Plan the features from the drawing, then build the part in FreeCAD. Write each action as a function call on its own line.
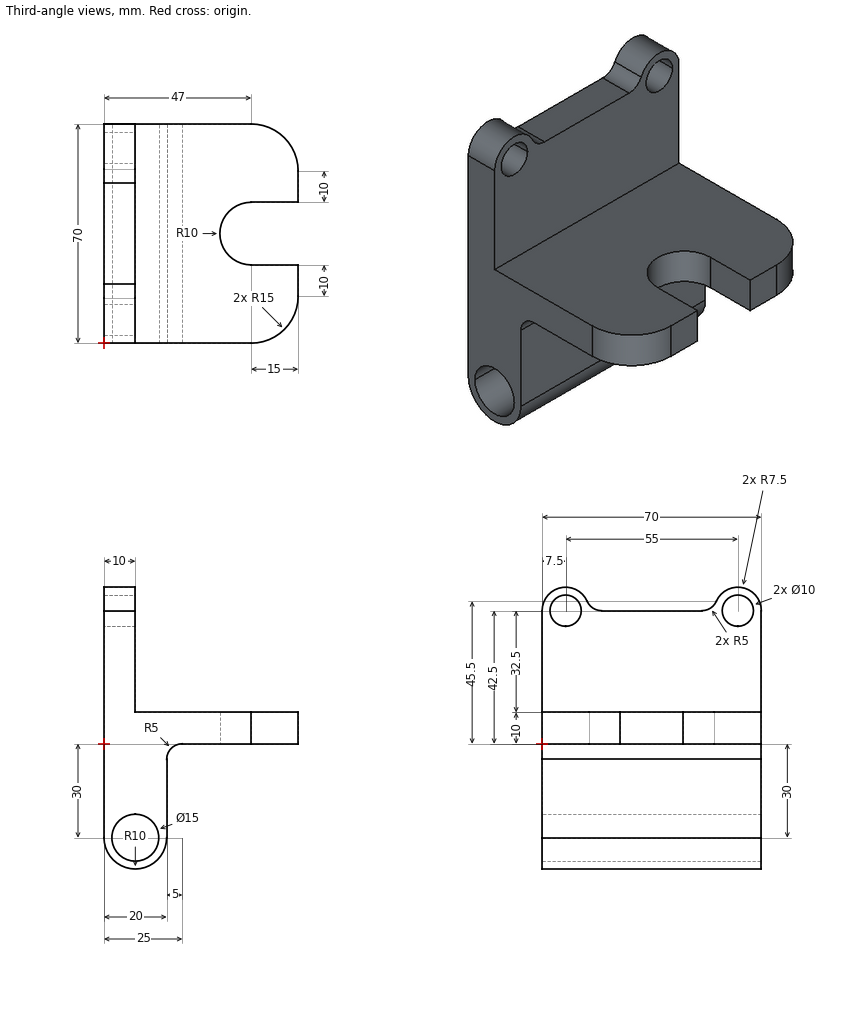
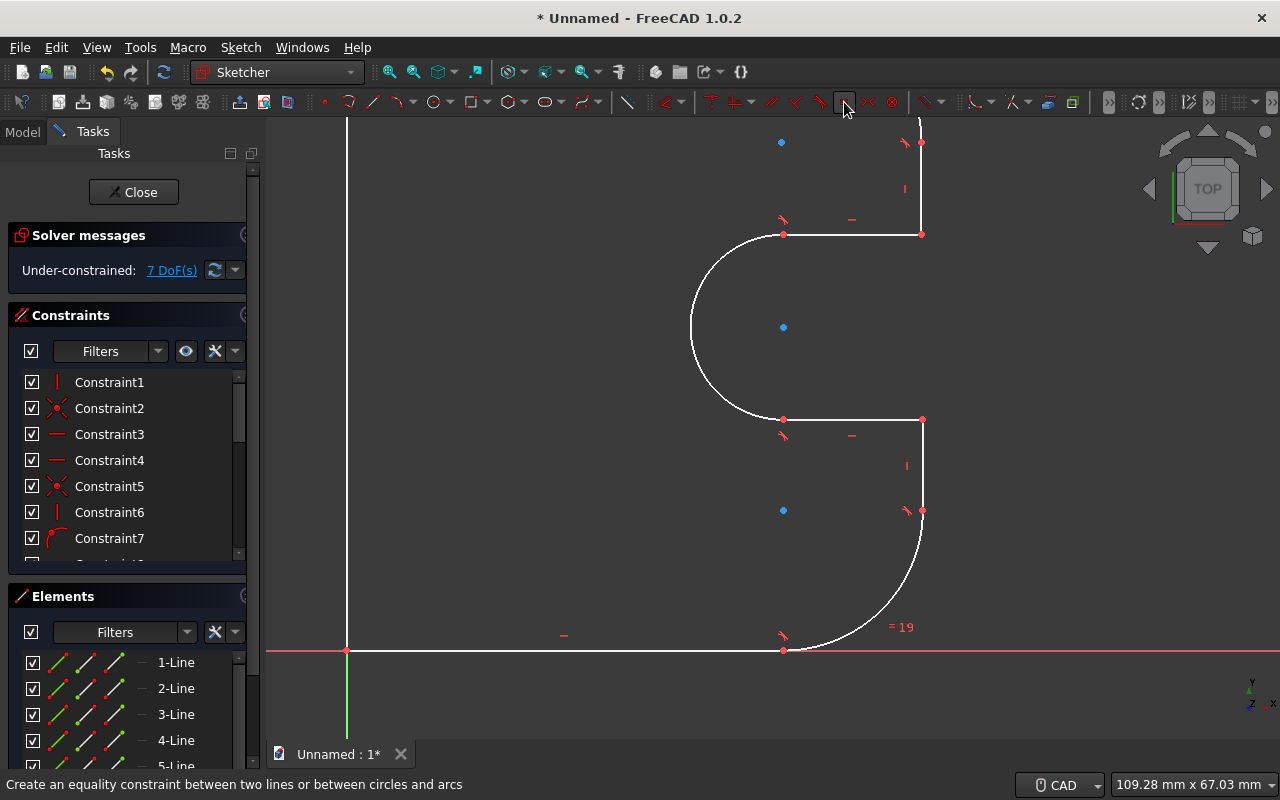
click(666, 102)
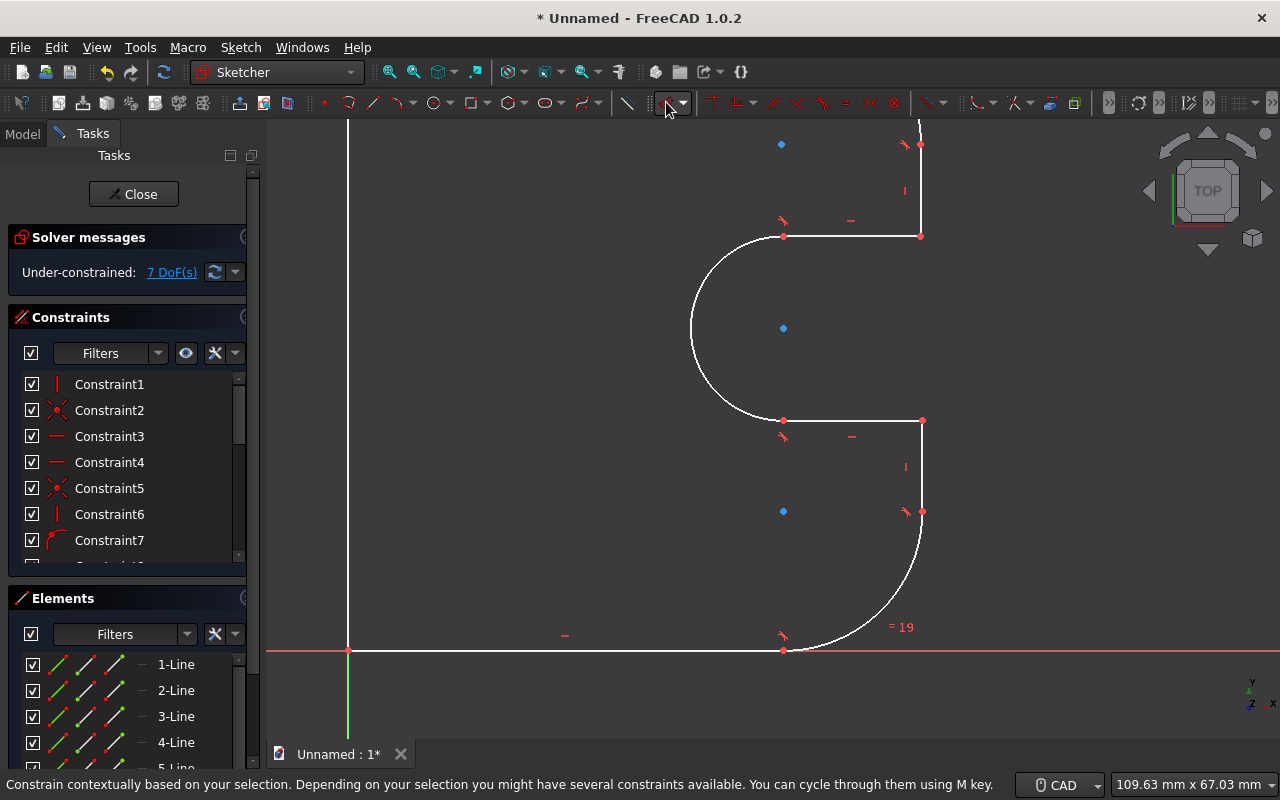
click(708, 274)
click(682, 255)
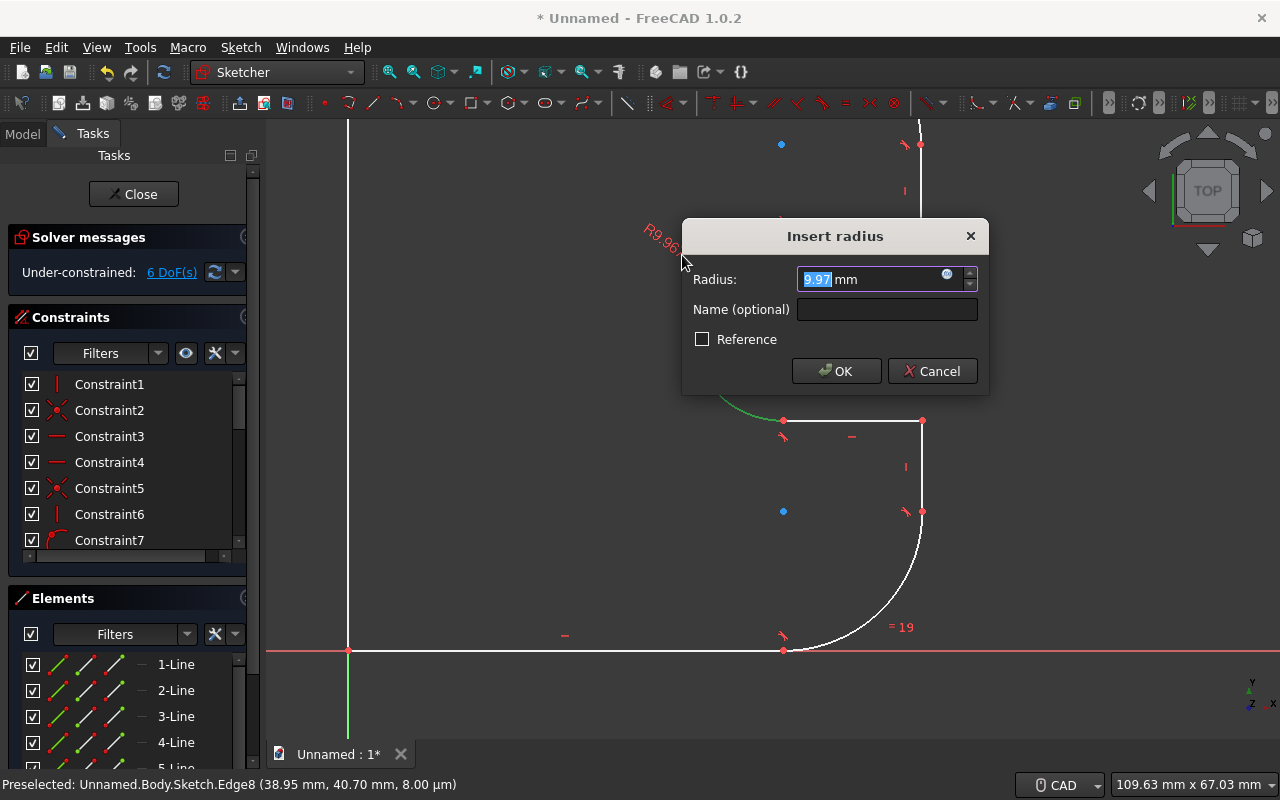
text(10)
key(Return)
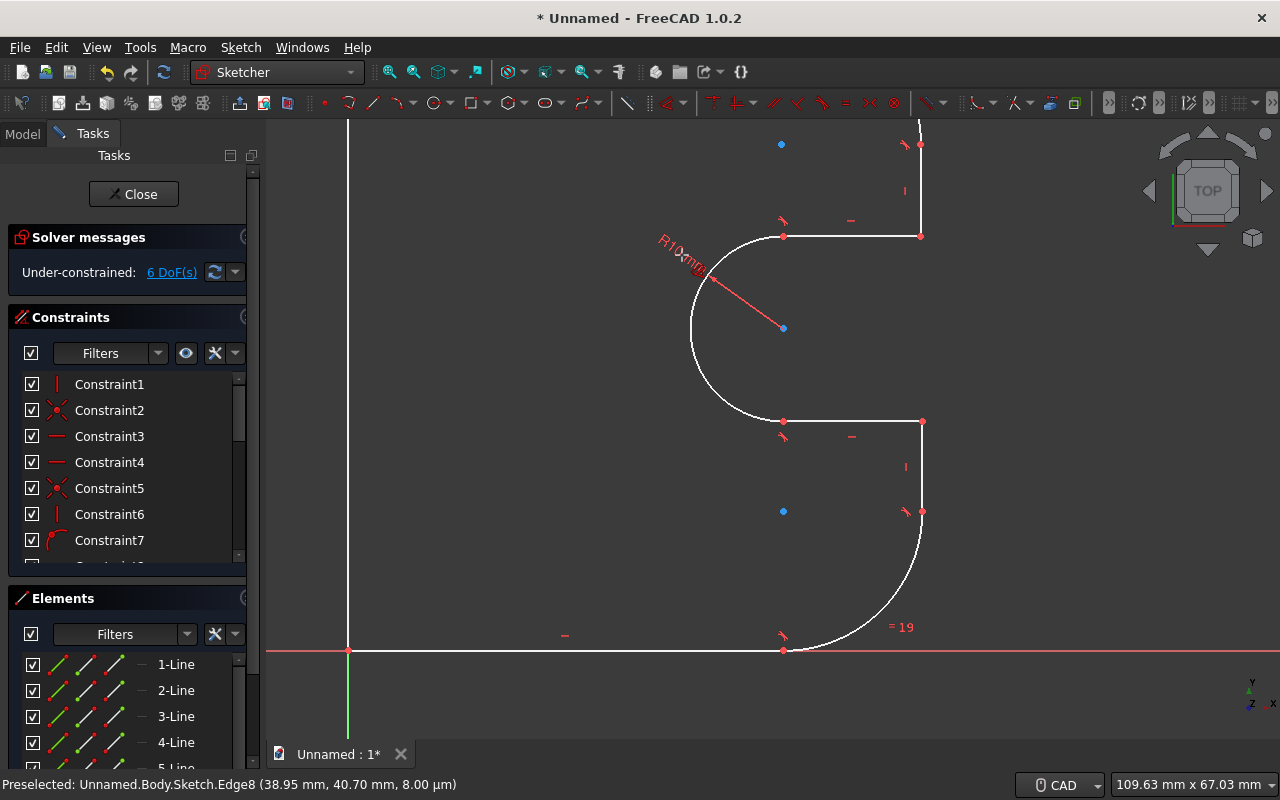
scroll(846, 636, down, 2)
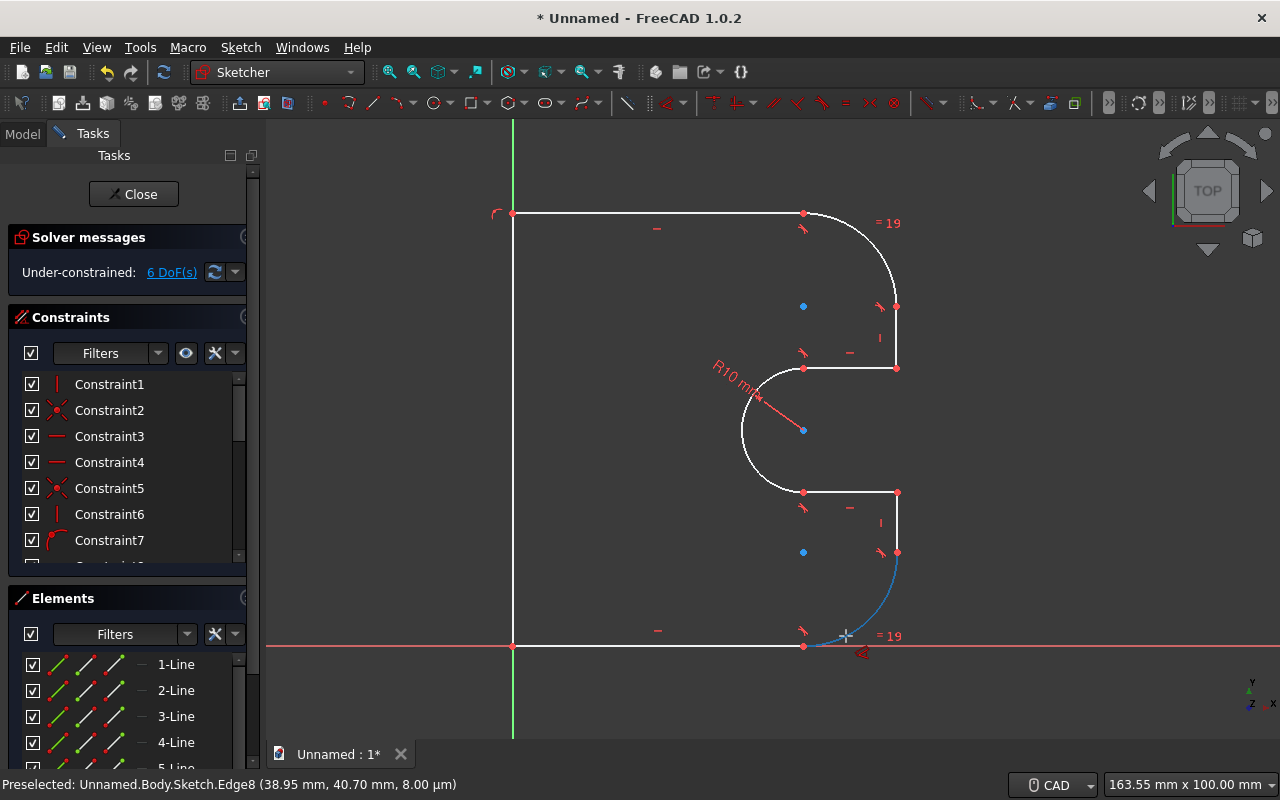
click(886, 264)
click(914, 249)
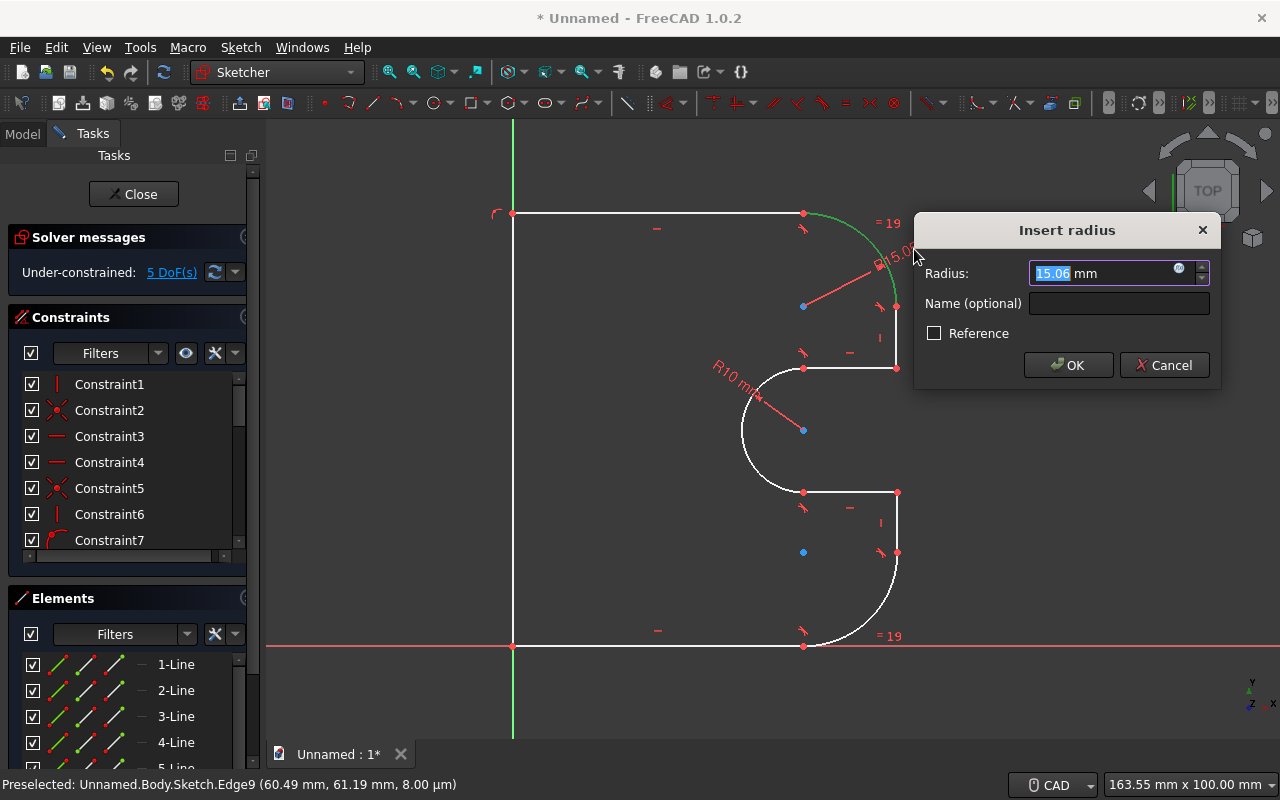
text(15)
key(Return)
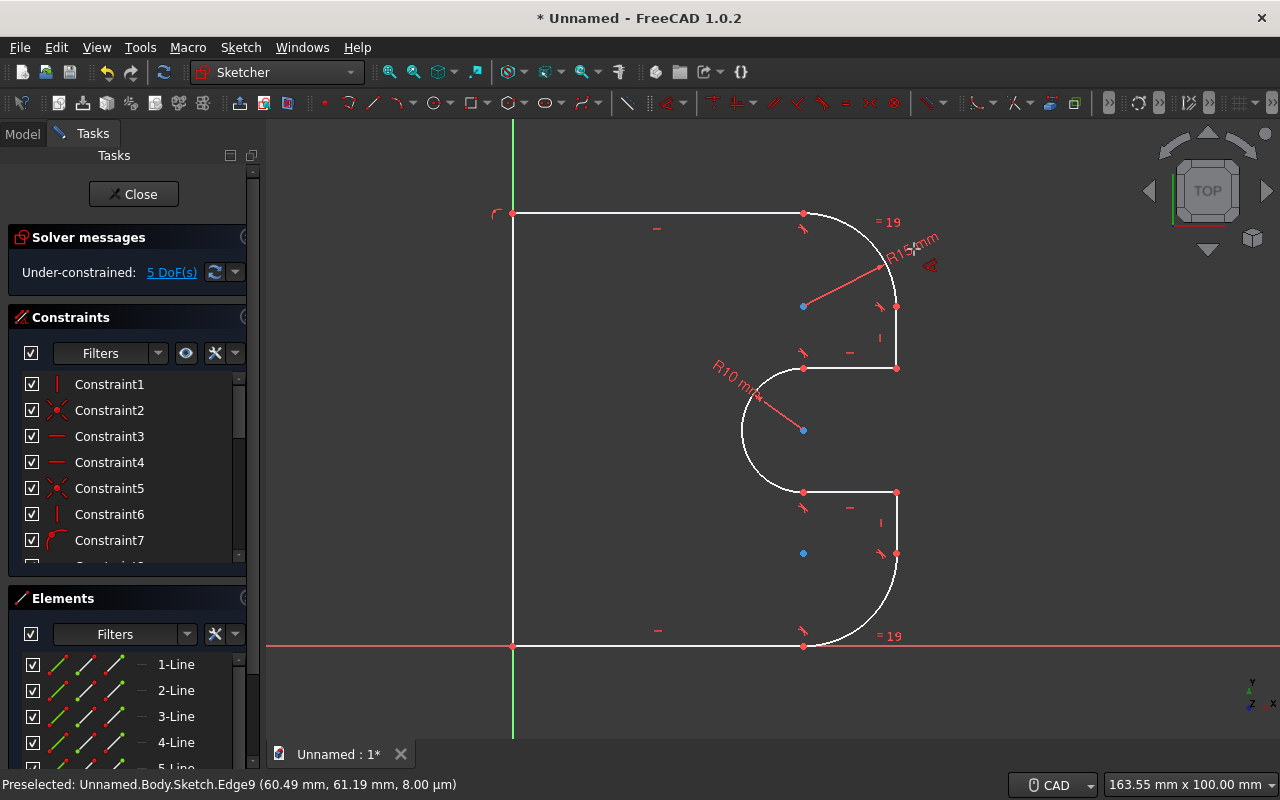
click(897, 535)
click(931, 523)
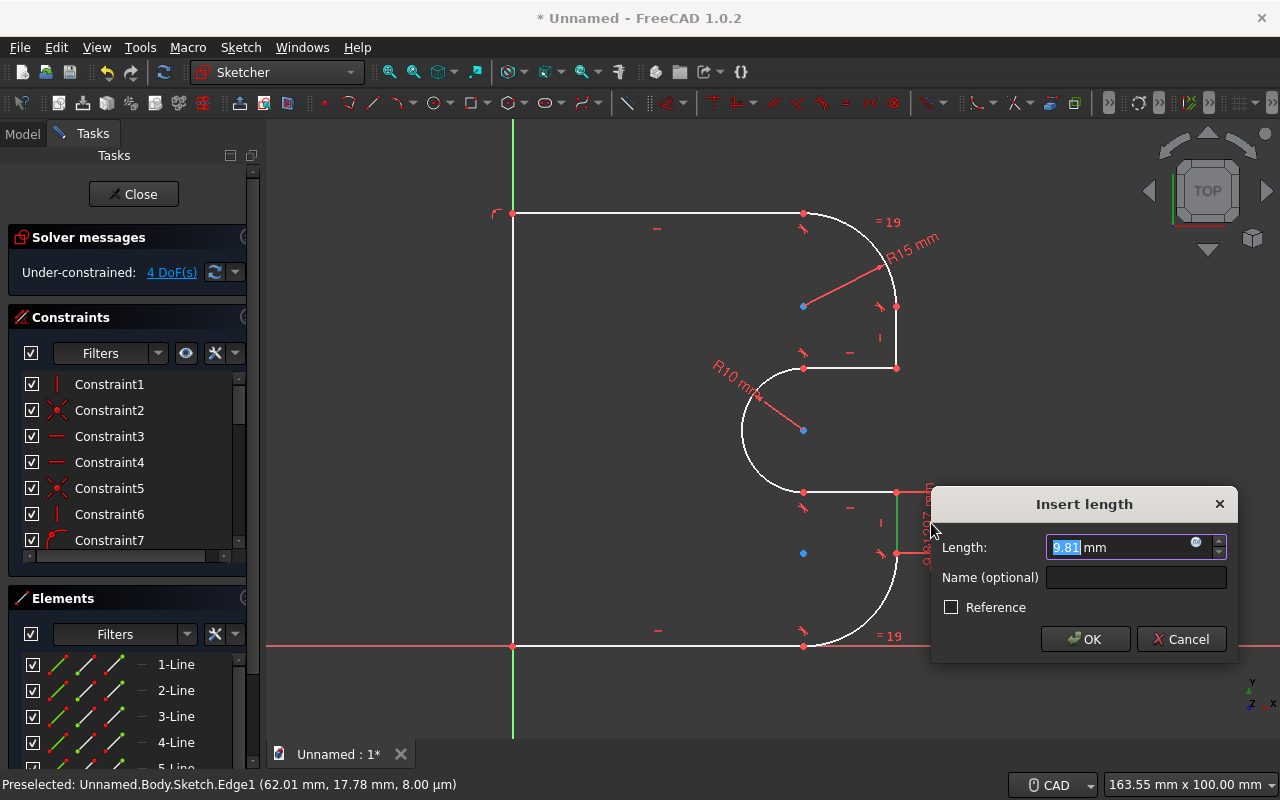
text(10)
key(Return)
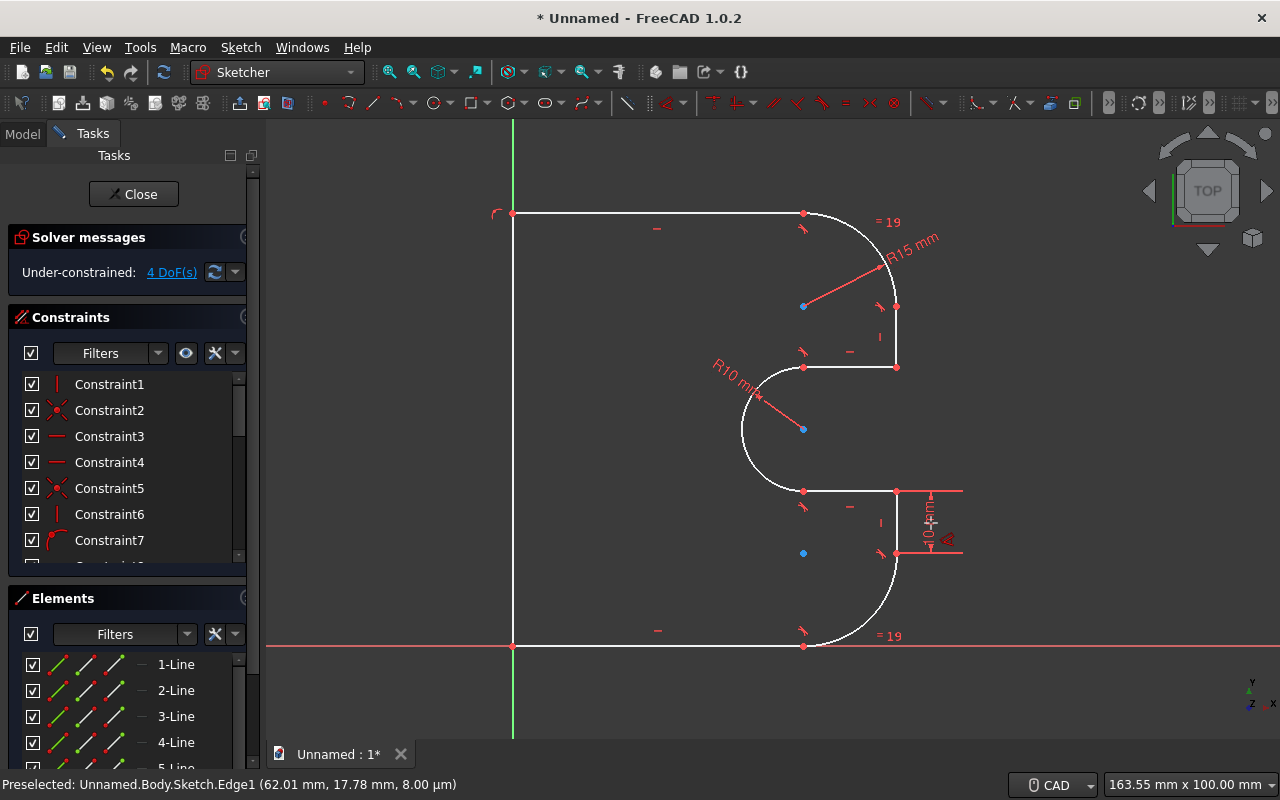
click(869, 491)
click(850, 525)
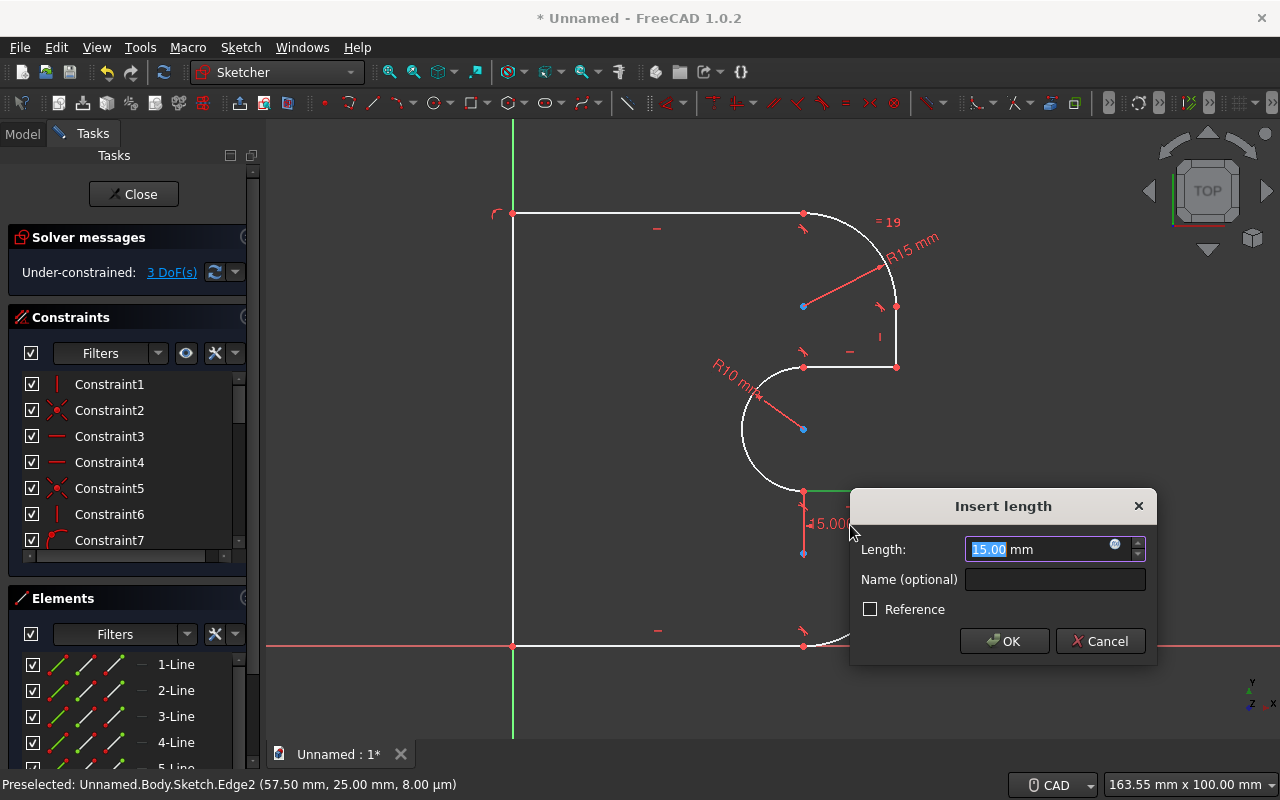
text(15)
key(Return)